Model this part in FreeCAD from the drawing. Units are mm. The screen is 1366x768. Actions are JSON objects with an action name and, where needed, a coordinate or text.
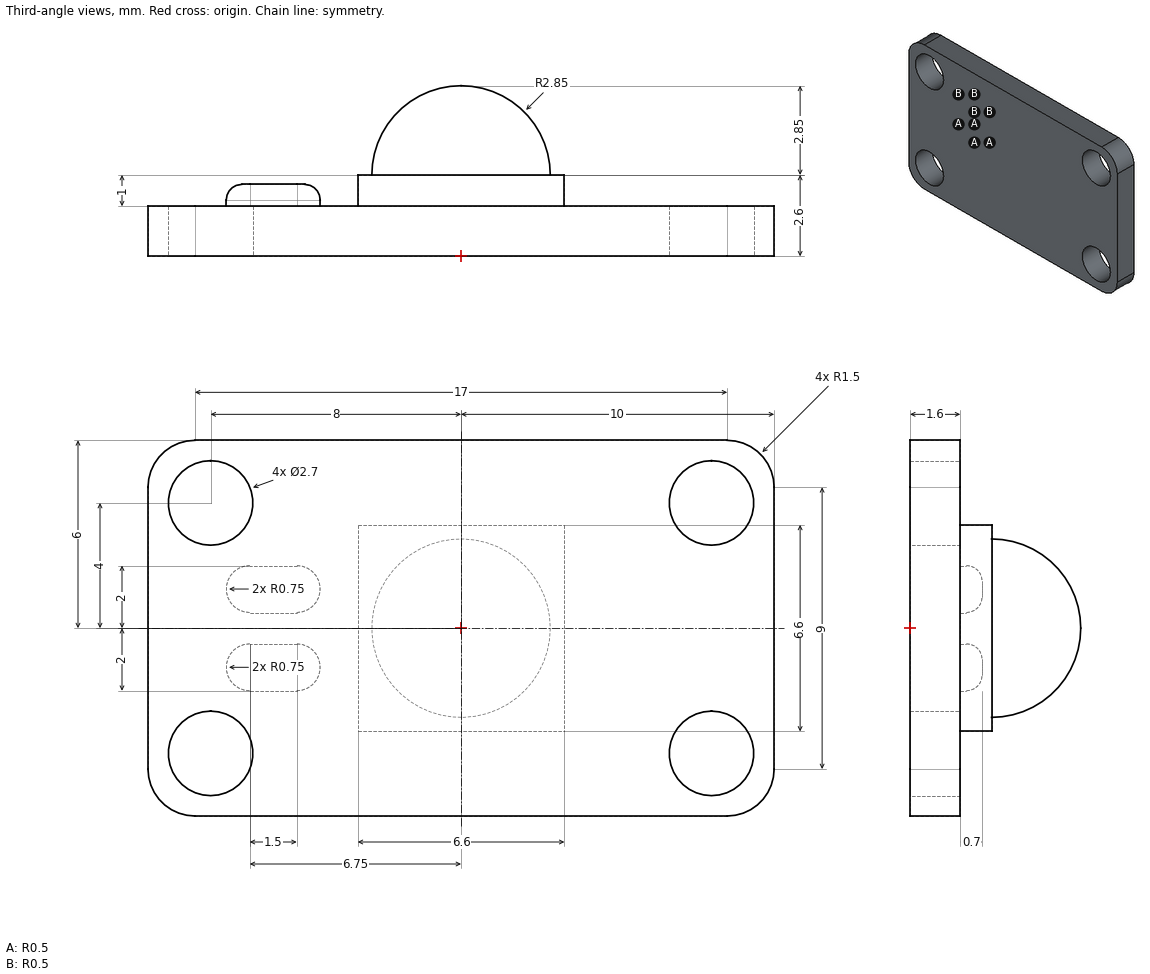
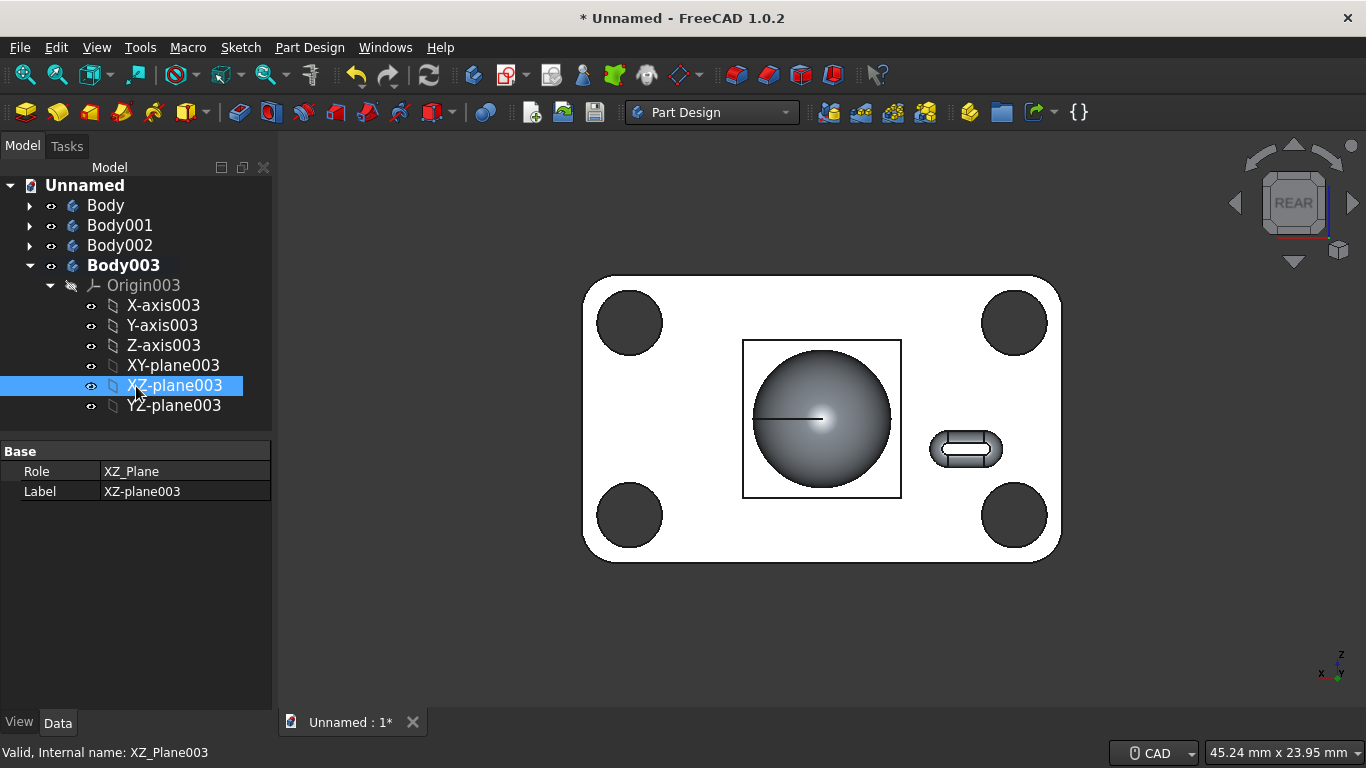
{"action": "left_click", "coordinate": [680, 76]}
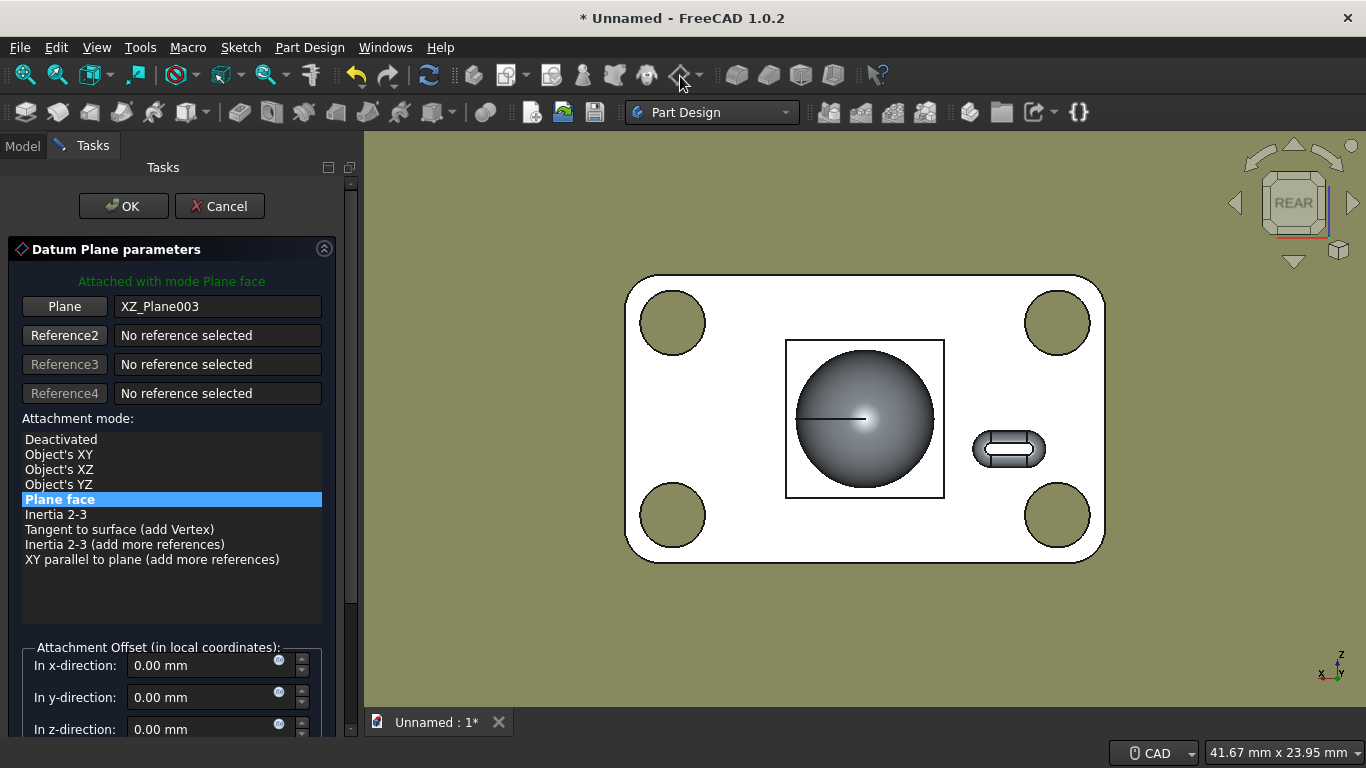
{"action": "scroll", "coordinate": [351, 456], "scroll_direction": "down", "scroll_amount": 2}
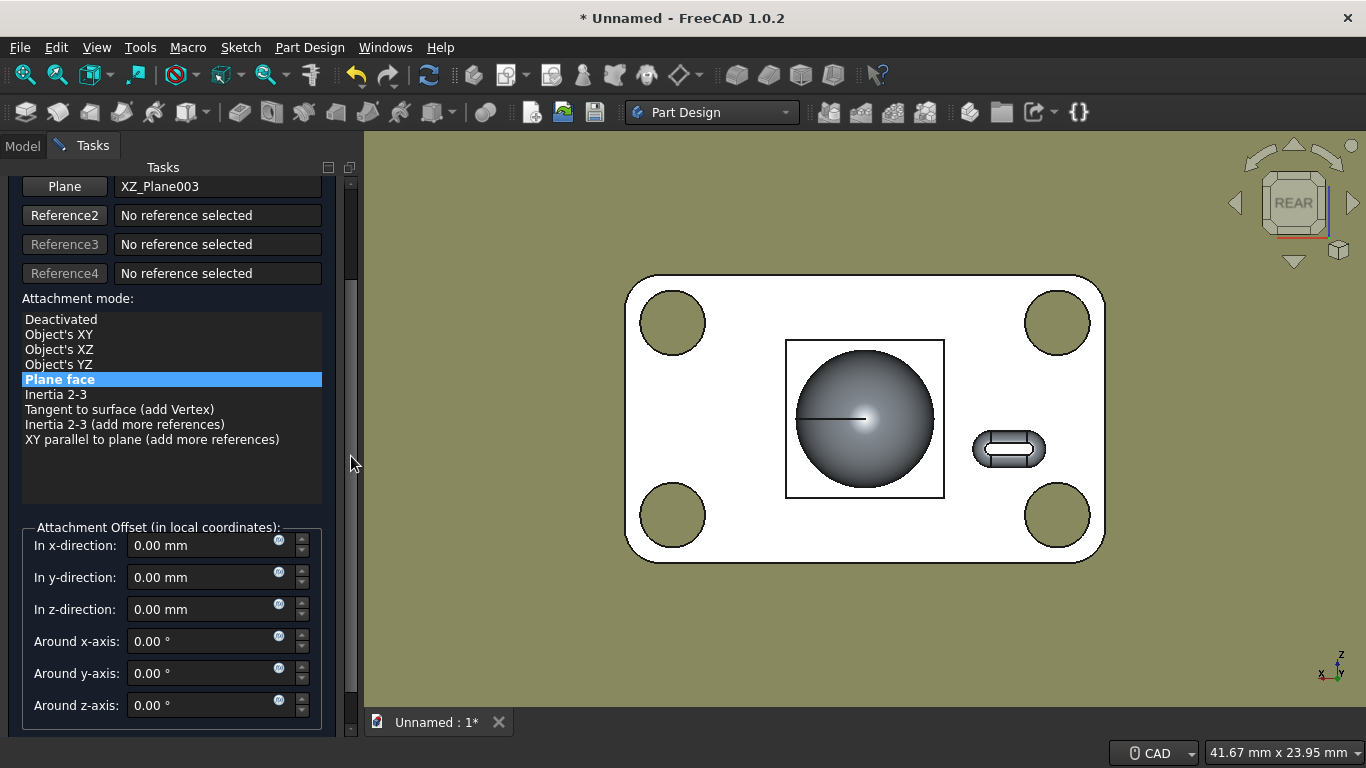
{"action": "triple_click", "coordinate": [210, 609]}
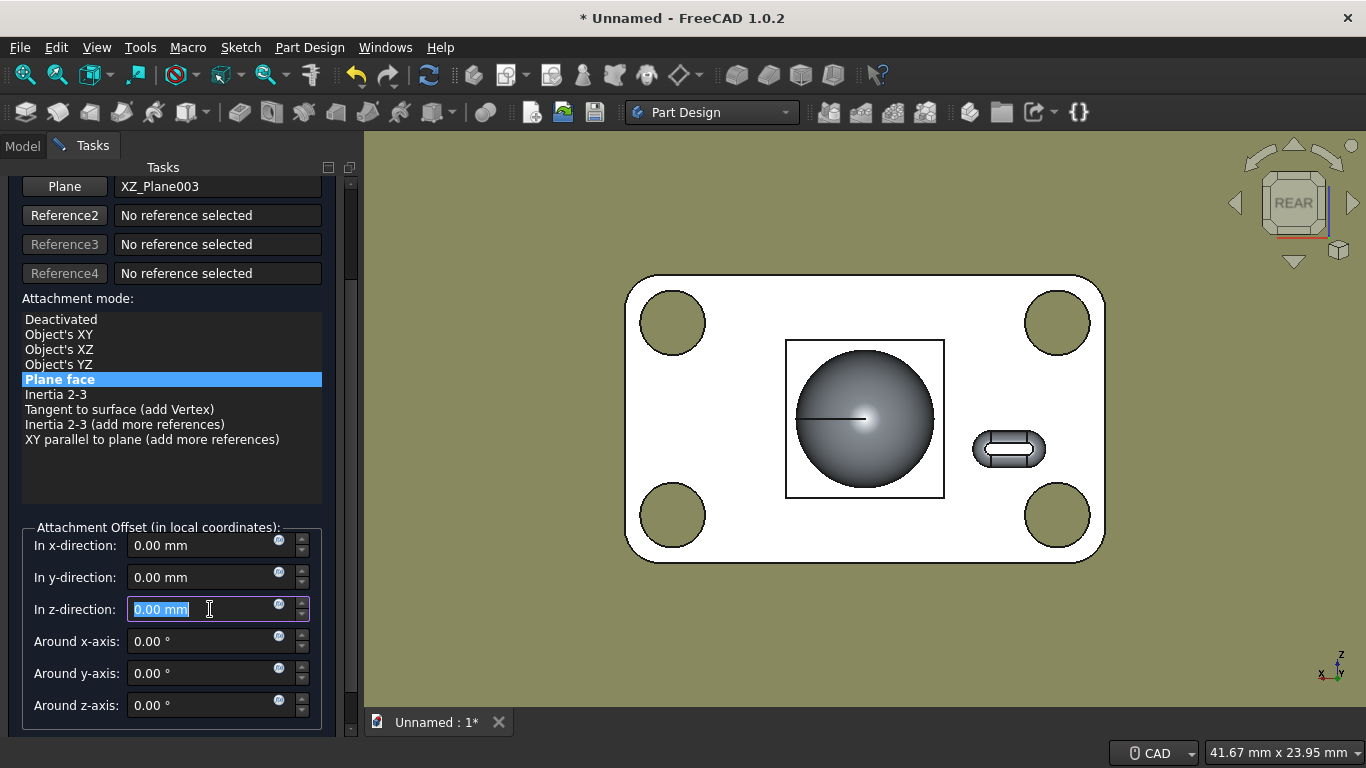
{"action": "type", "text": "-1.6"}
{"action": "key", "text": "Tab"}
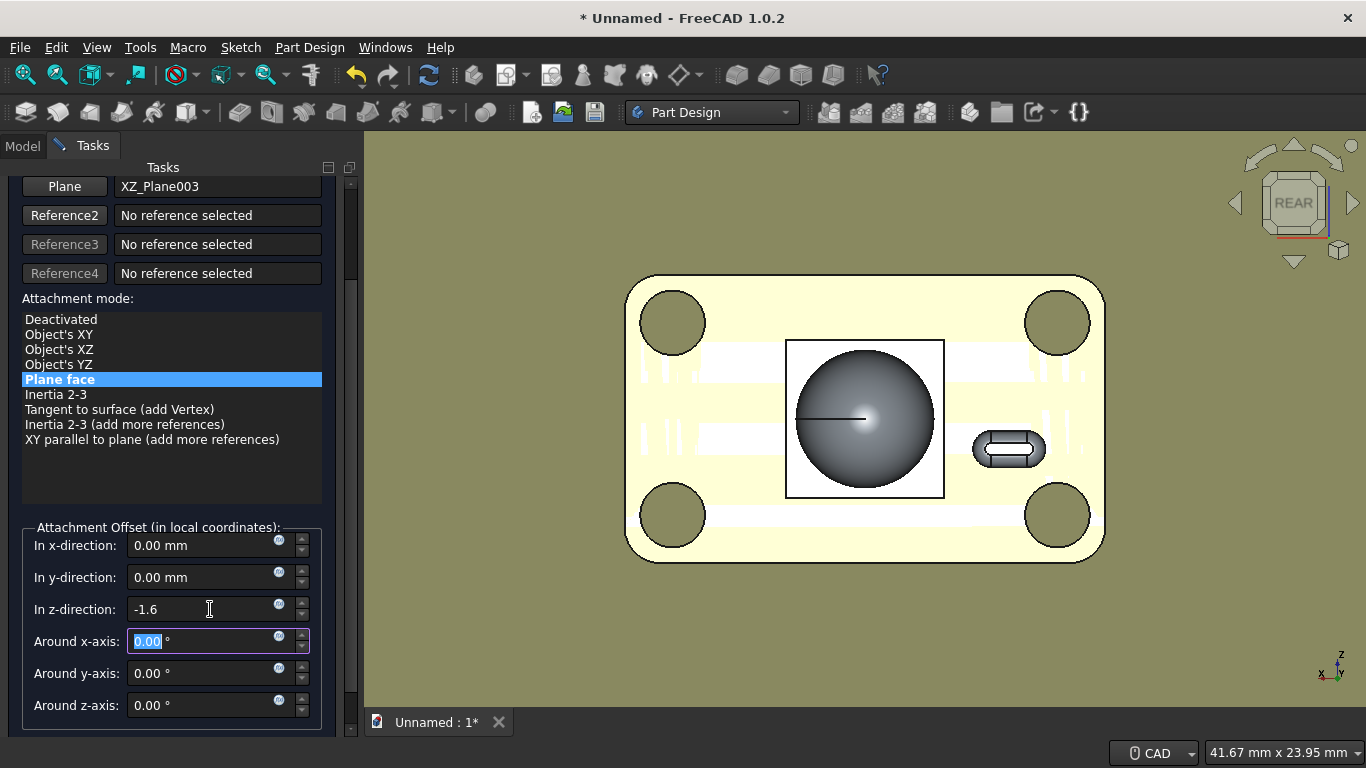
{"action": "scroll", "coordinate": [351, 456], "scroll_direction": "up", "scroll_amount": 3}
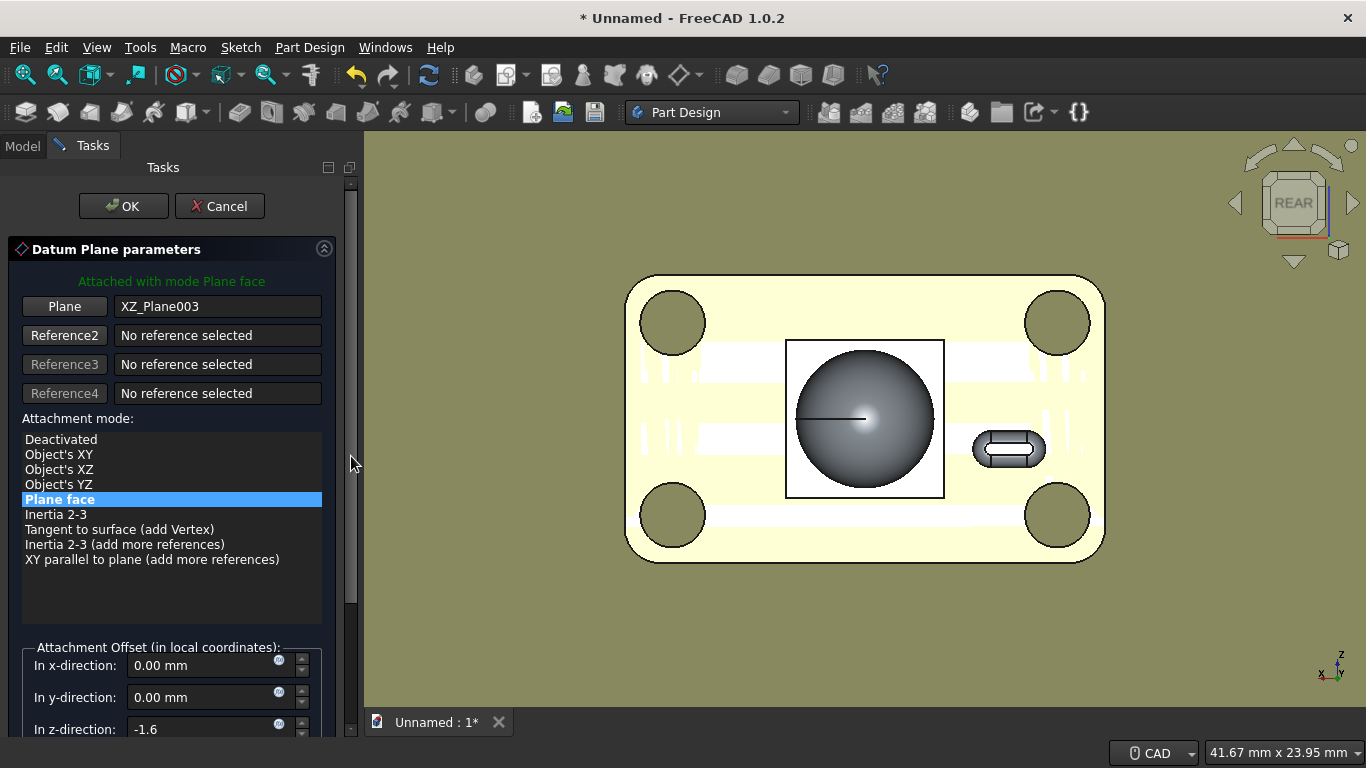
{"action": "left_click", "coordinate": [124, 206]}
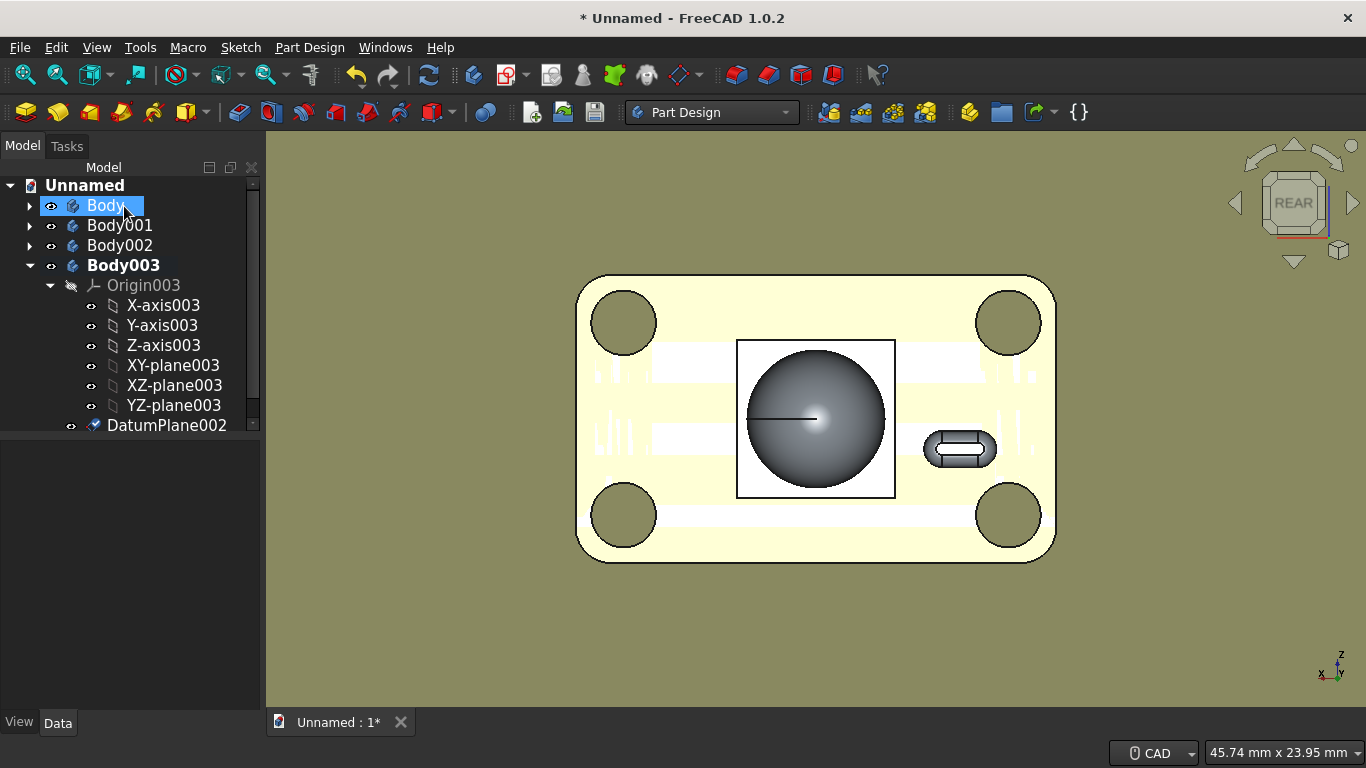
{"action": "left_click", "coordinate": [116, 426]}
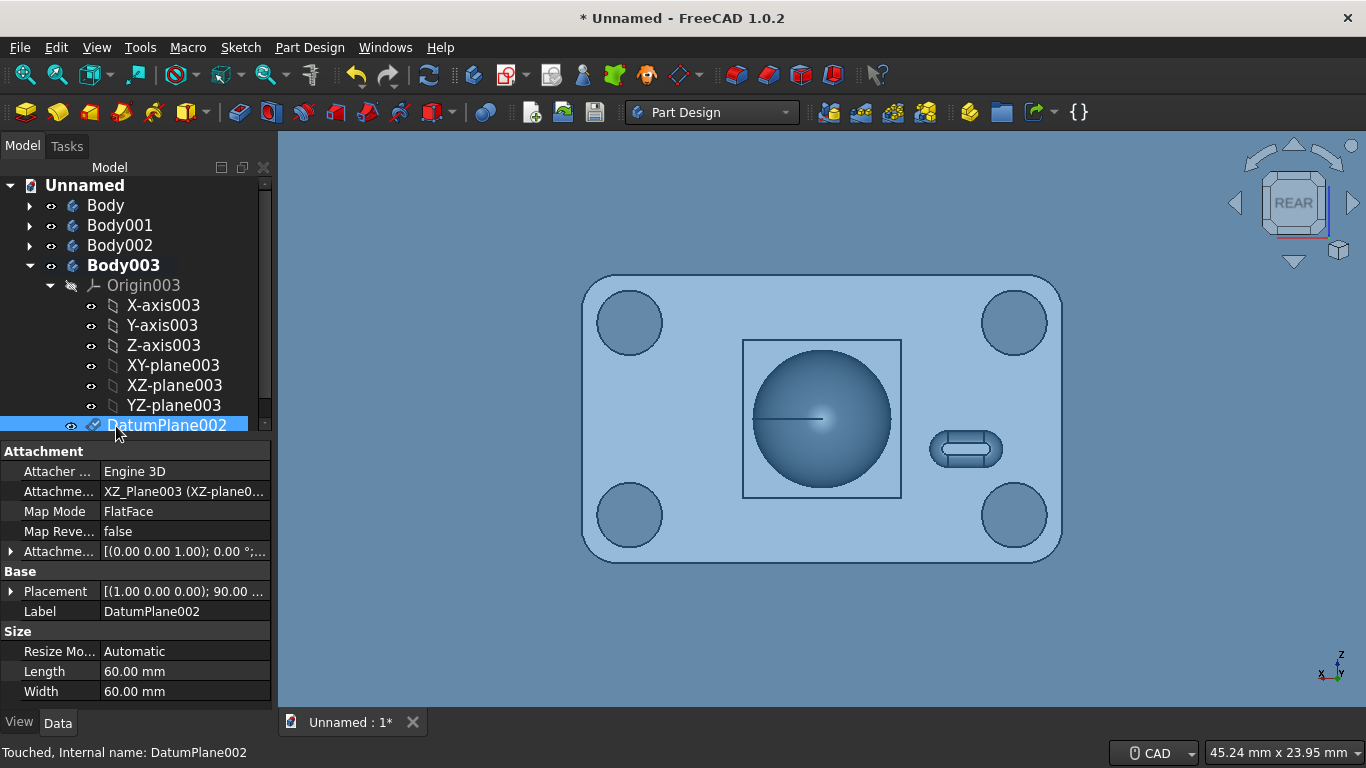
{"action": "left_click", "coordinate": [506, 76]}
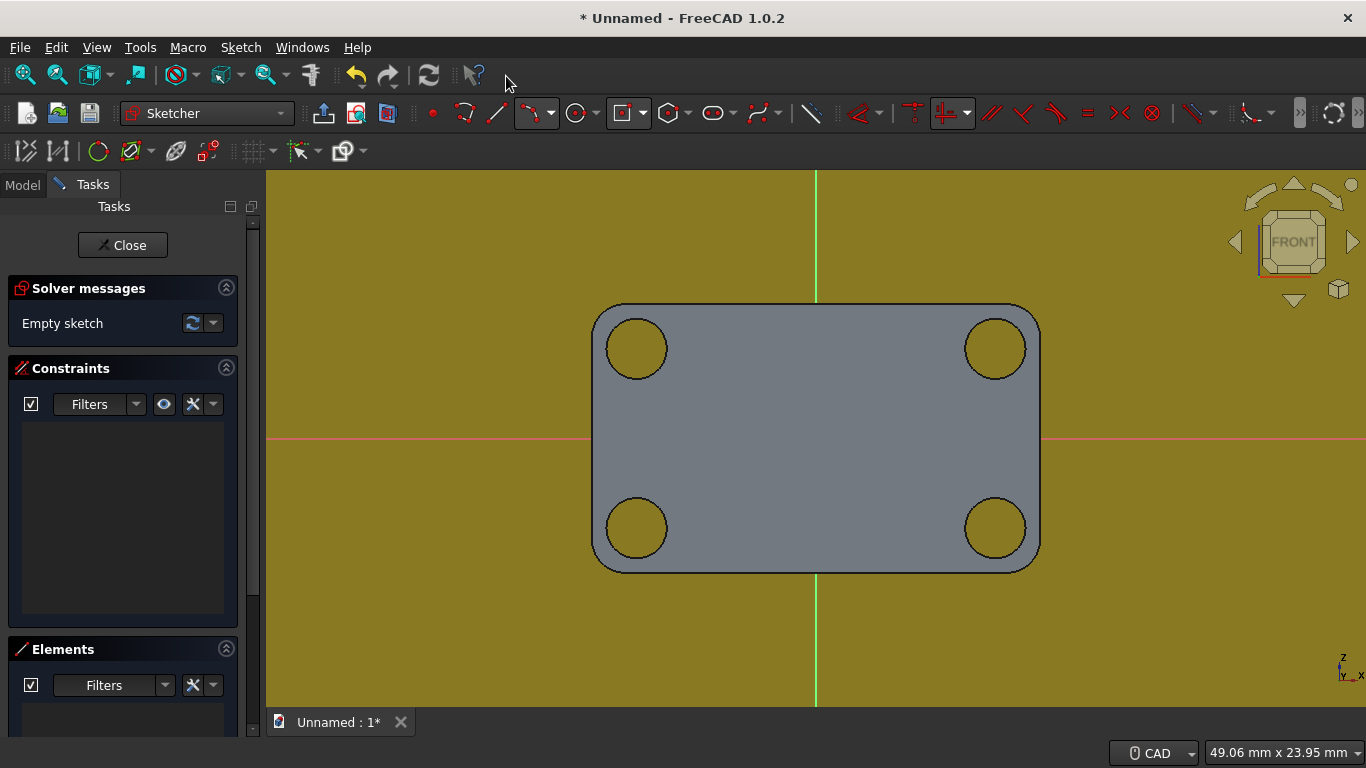
{"action": "scroll", "coordinate": [673, 407], "scroll_direction": "up", "scroll_amount": 11}